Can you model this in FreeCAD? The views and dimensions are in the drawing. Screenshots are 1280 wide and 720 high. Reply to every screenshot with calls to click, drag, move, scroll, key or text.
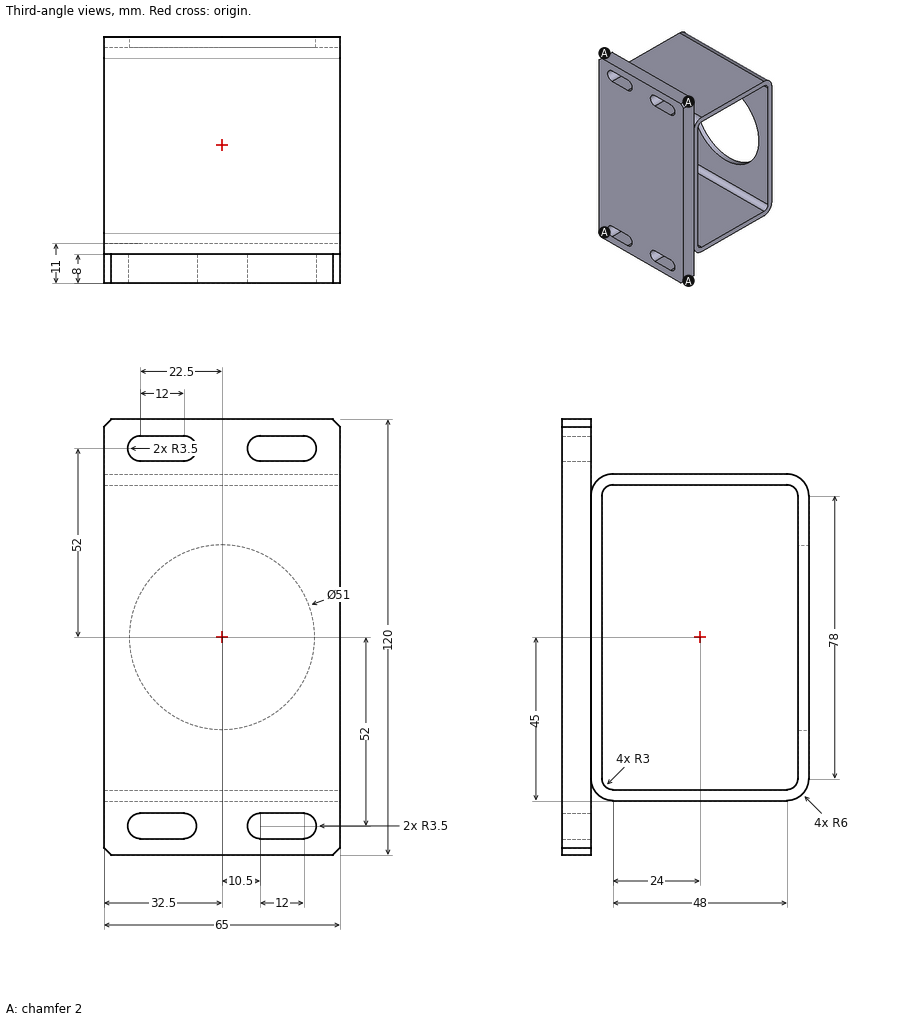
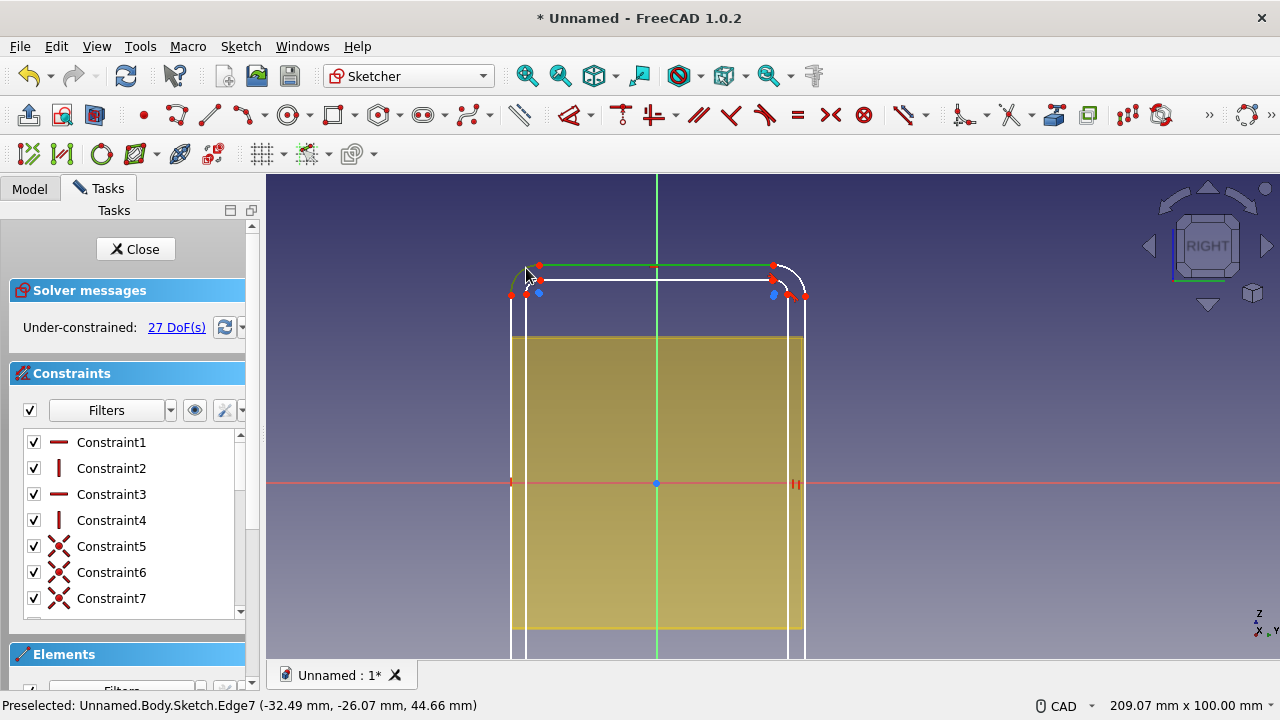
click(765, 116)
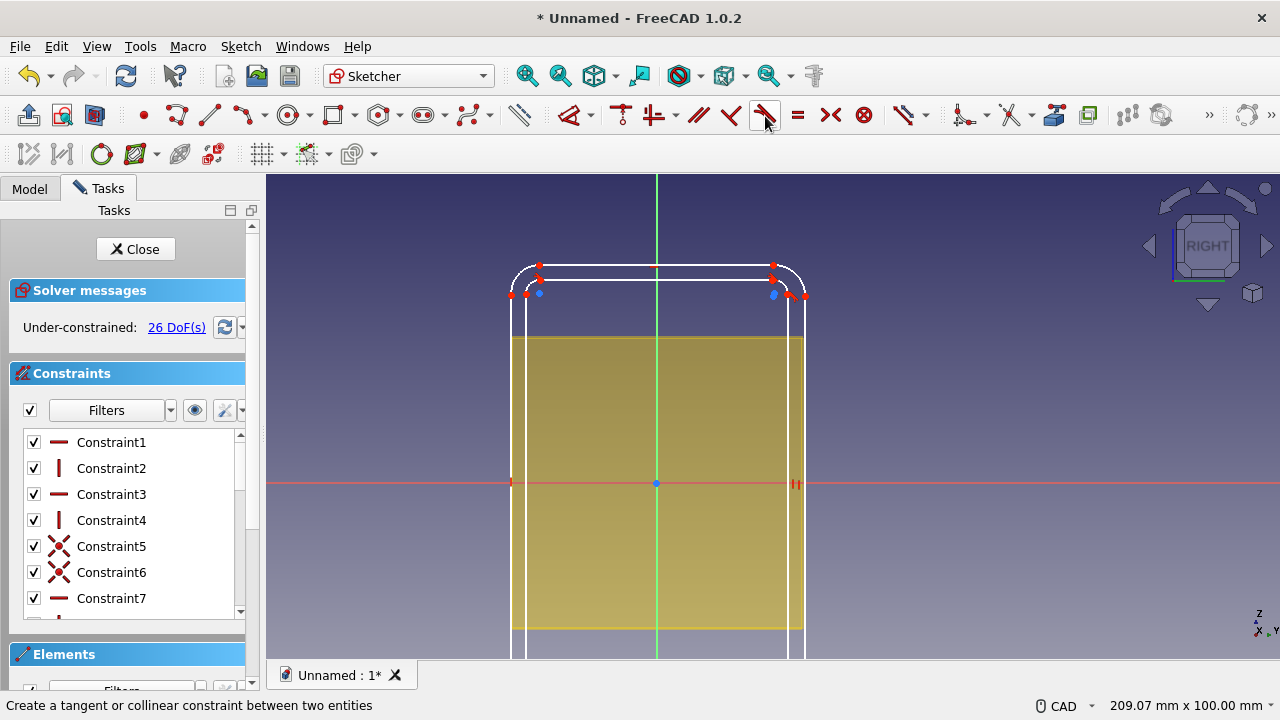
click(511, 409)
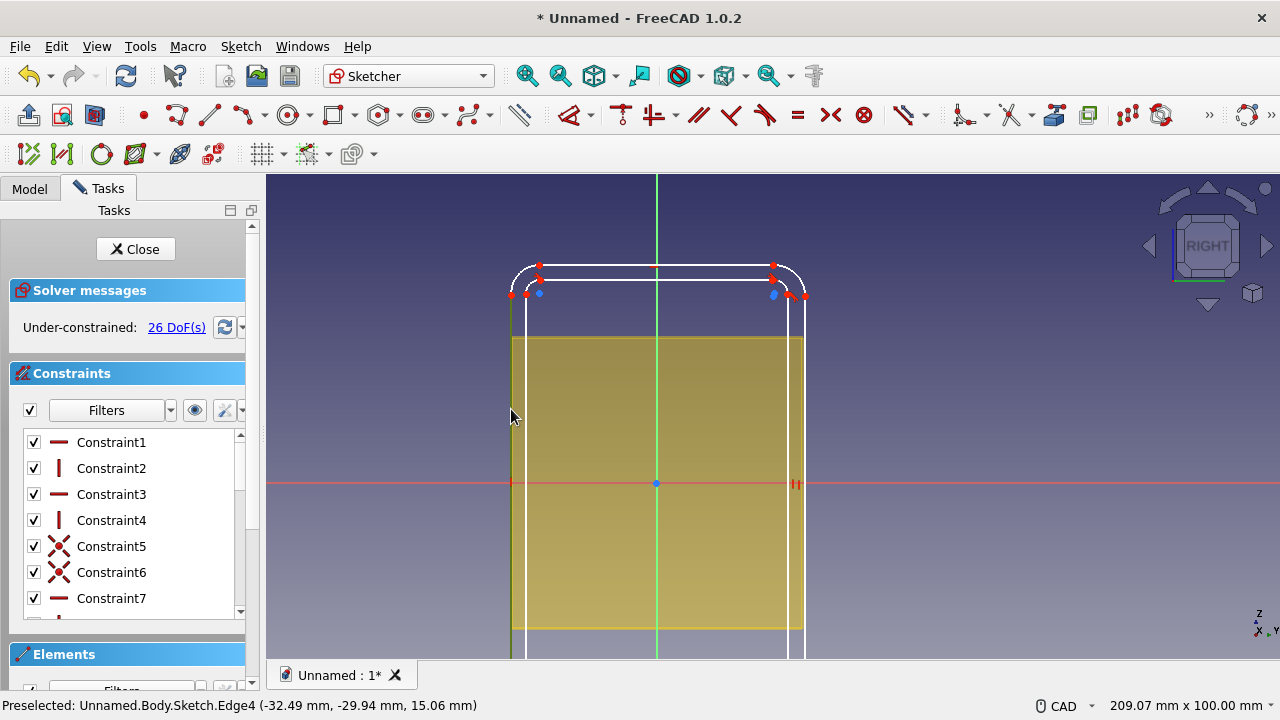
click(526, 269)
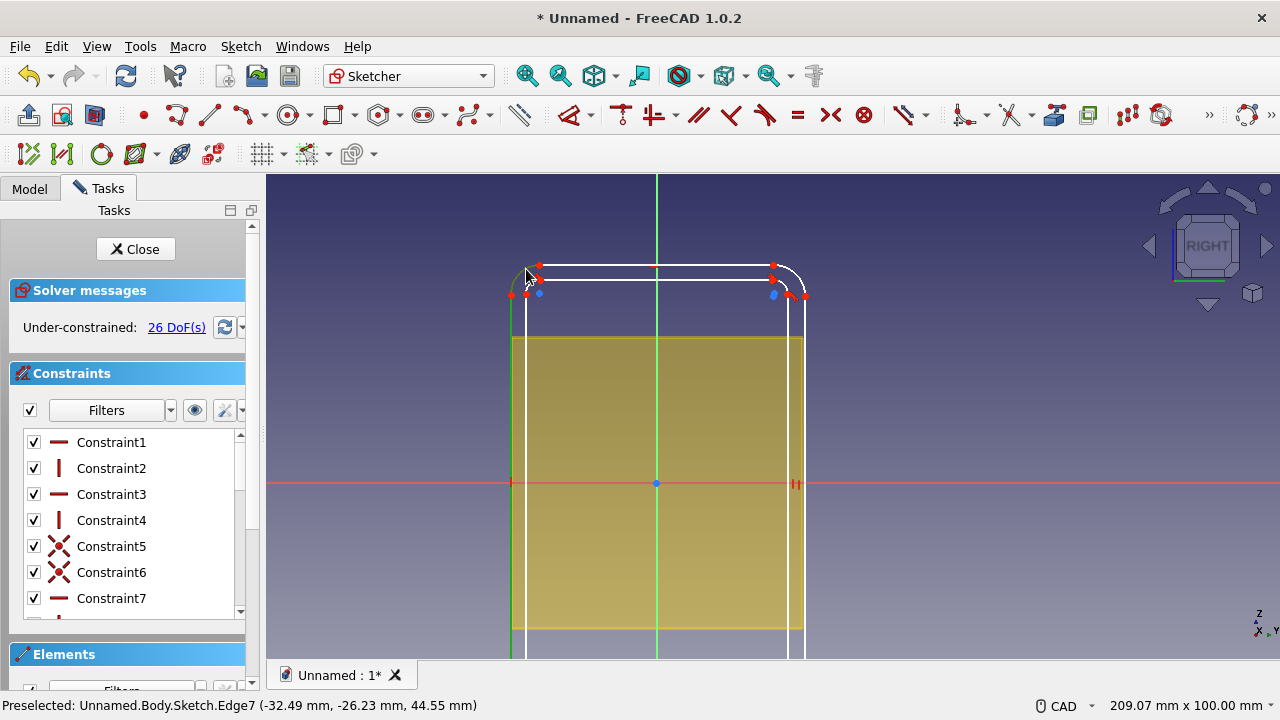
click(765, 116)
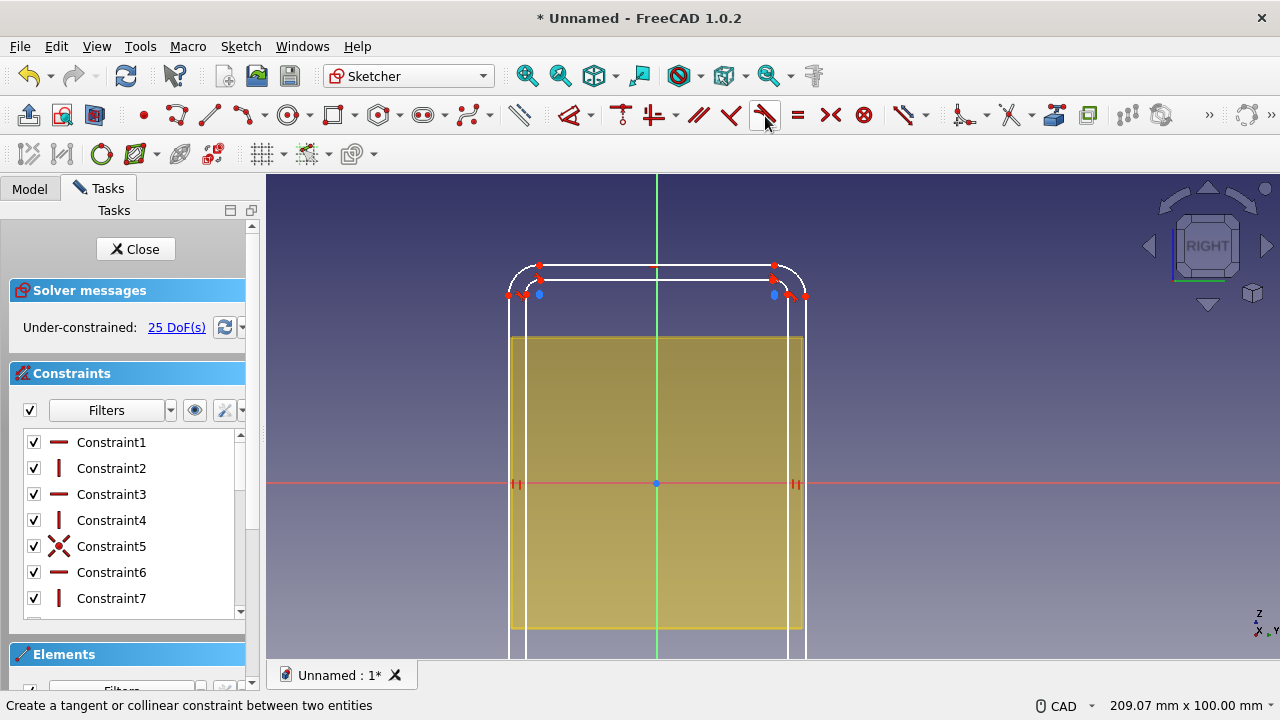
click(509, 409)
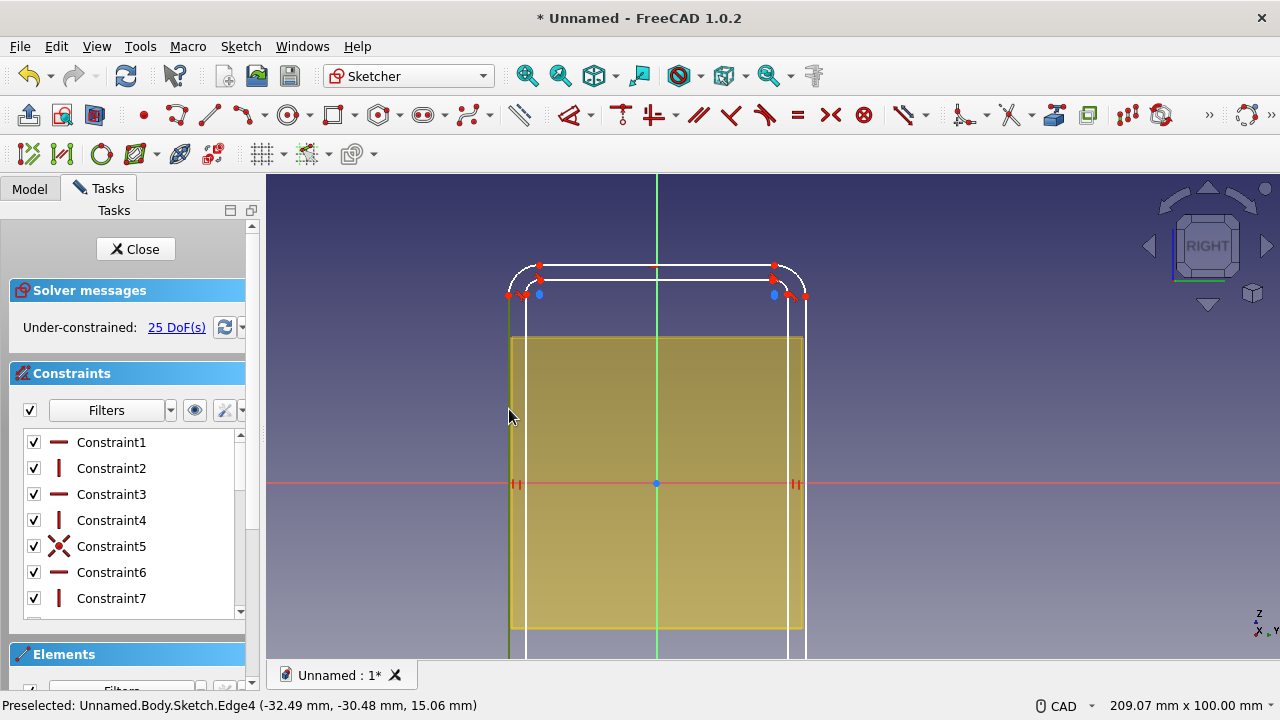
scroll(802, 281, down, 2)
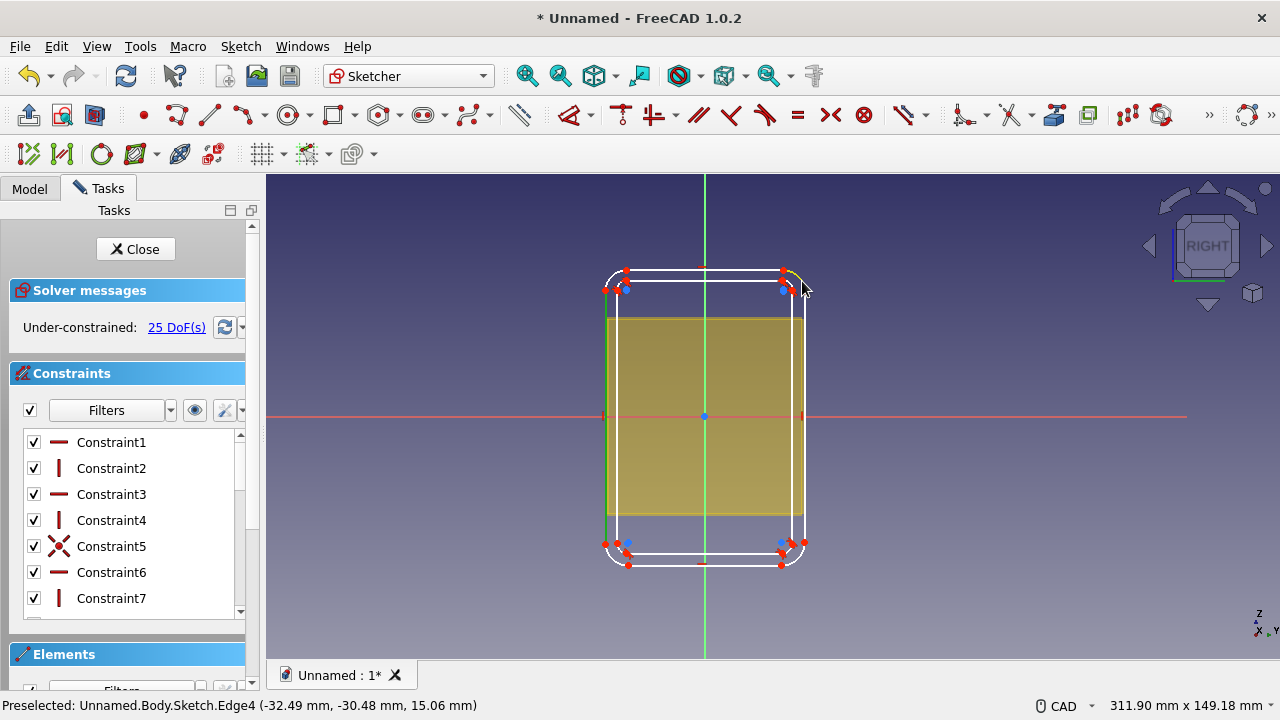
scroll(609, 554, up, 2)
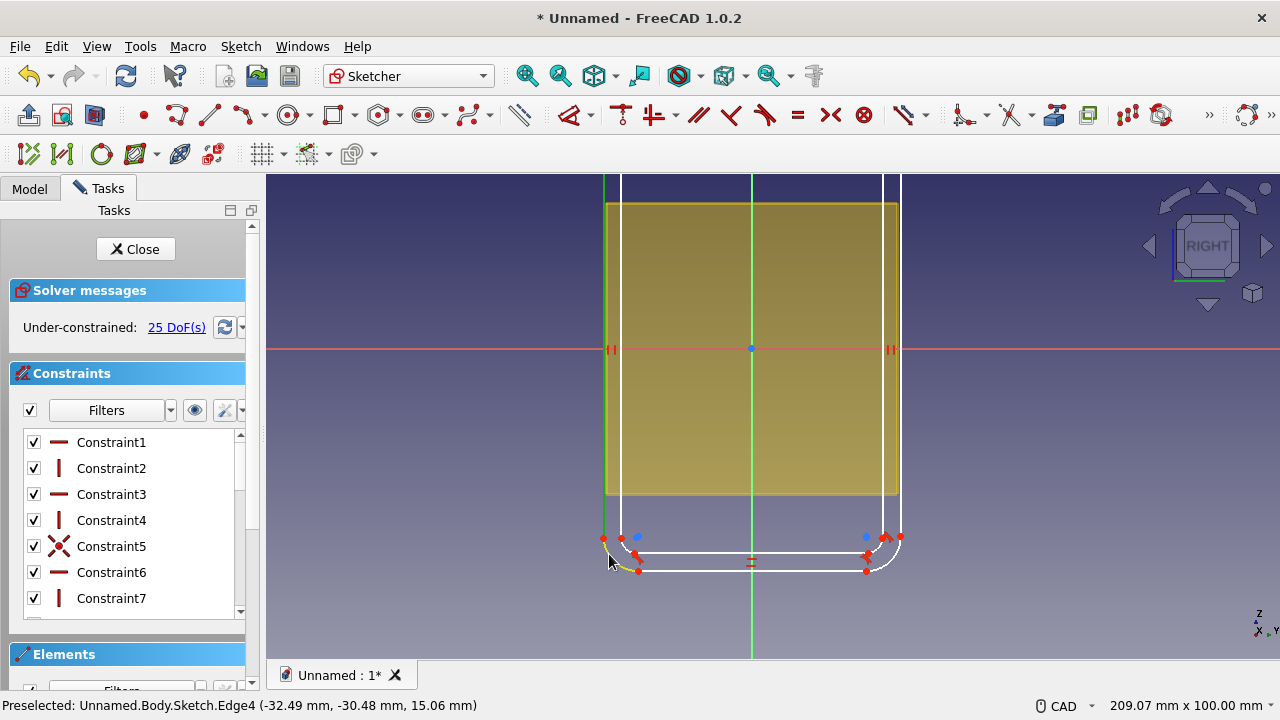
click(608, 554)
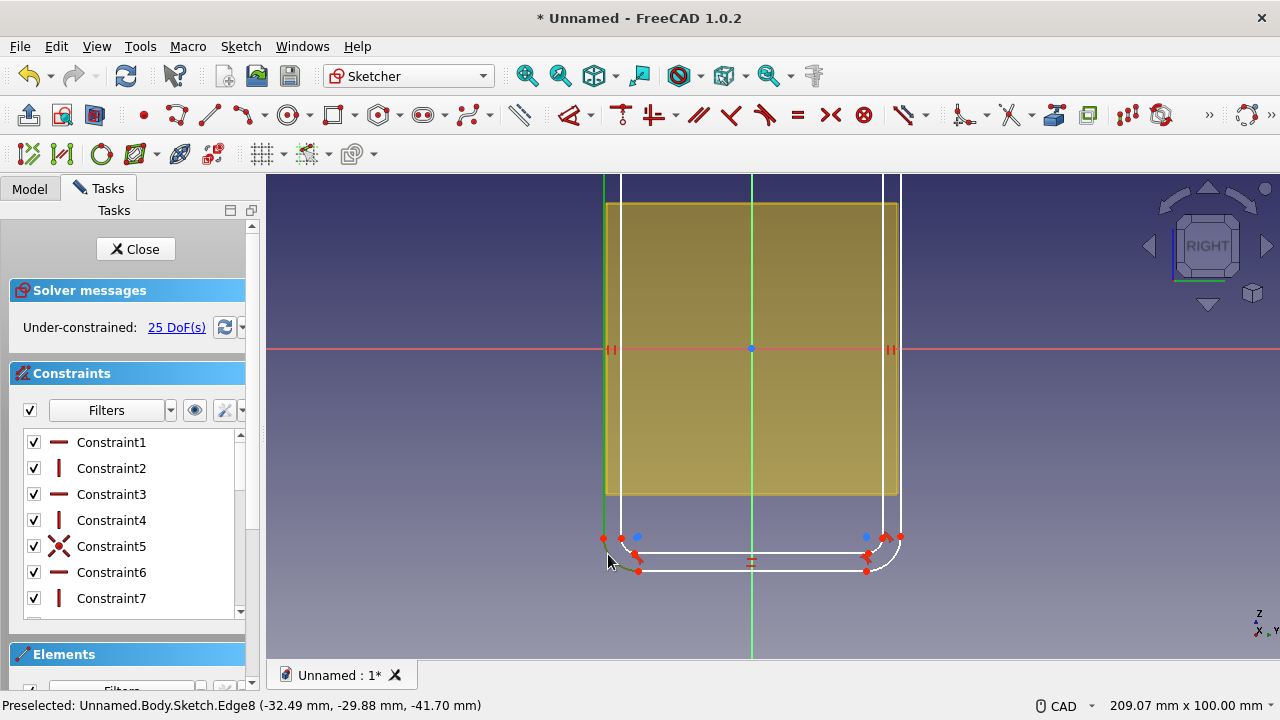
click(765, 116)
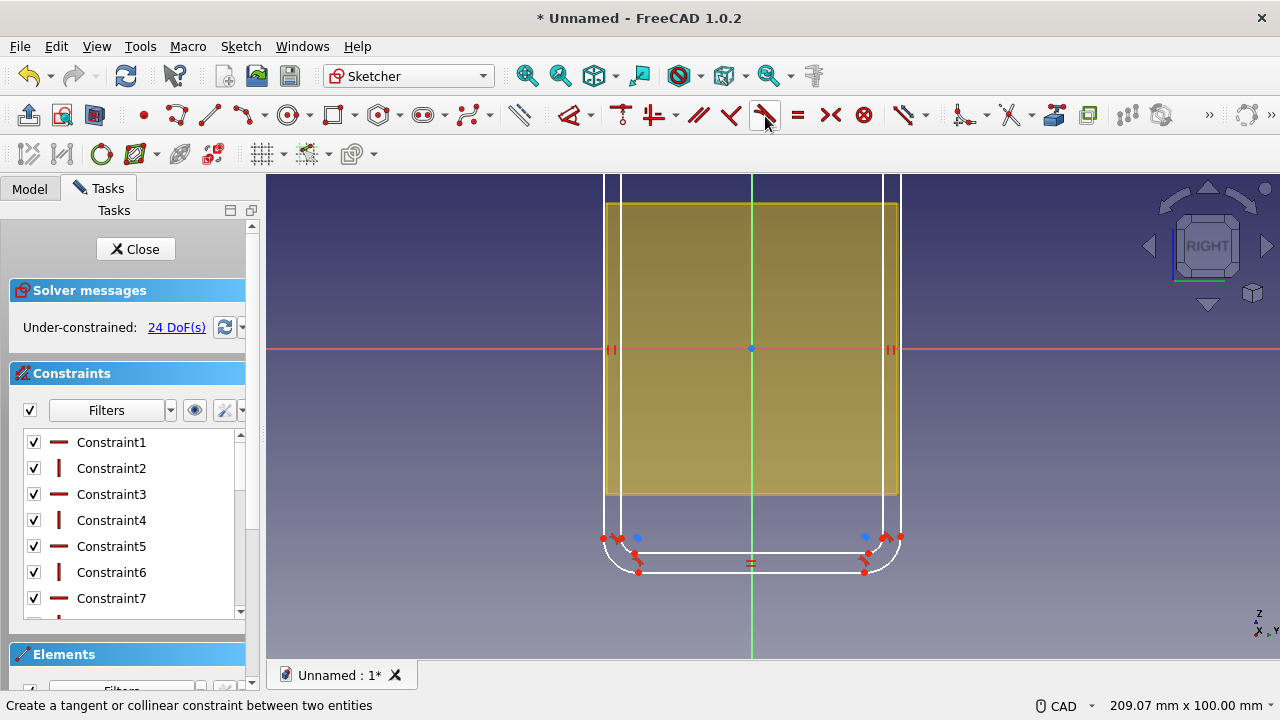
click(798, 553)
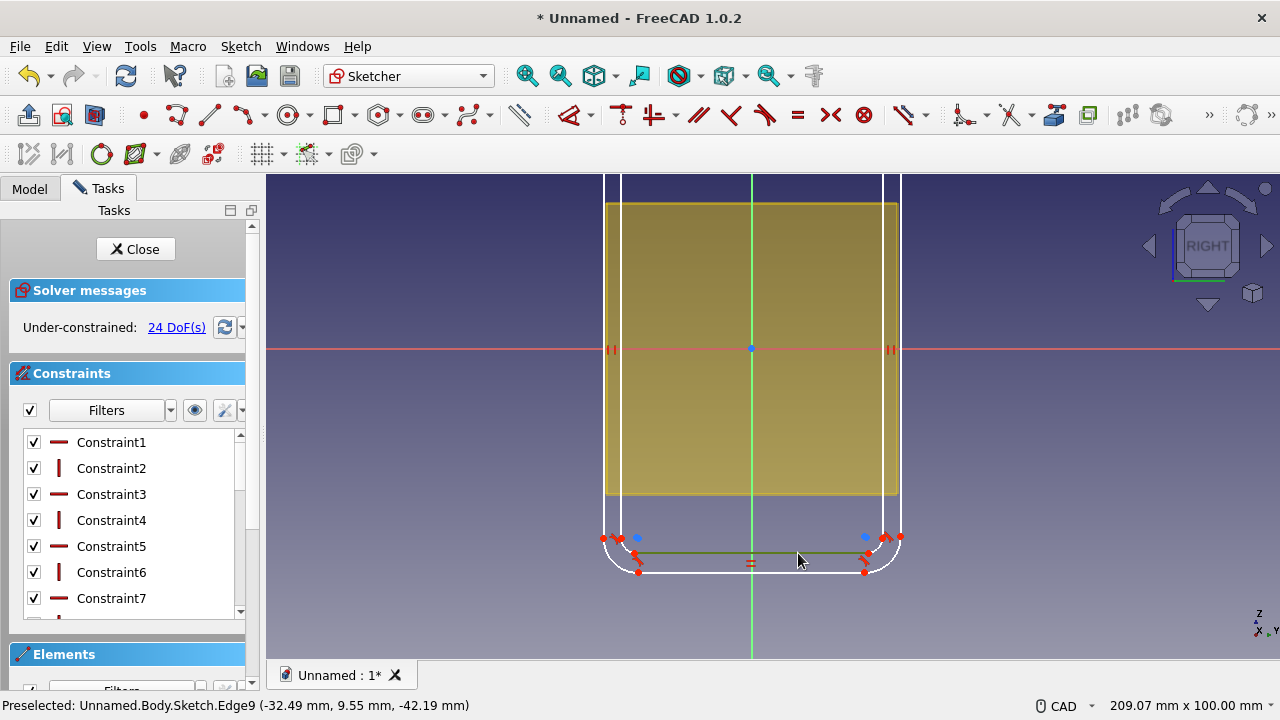
scroll(625, 548, up, 2)